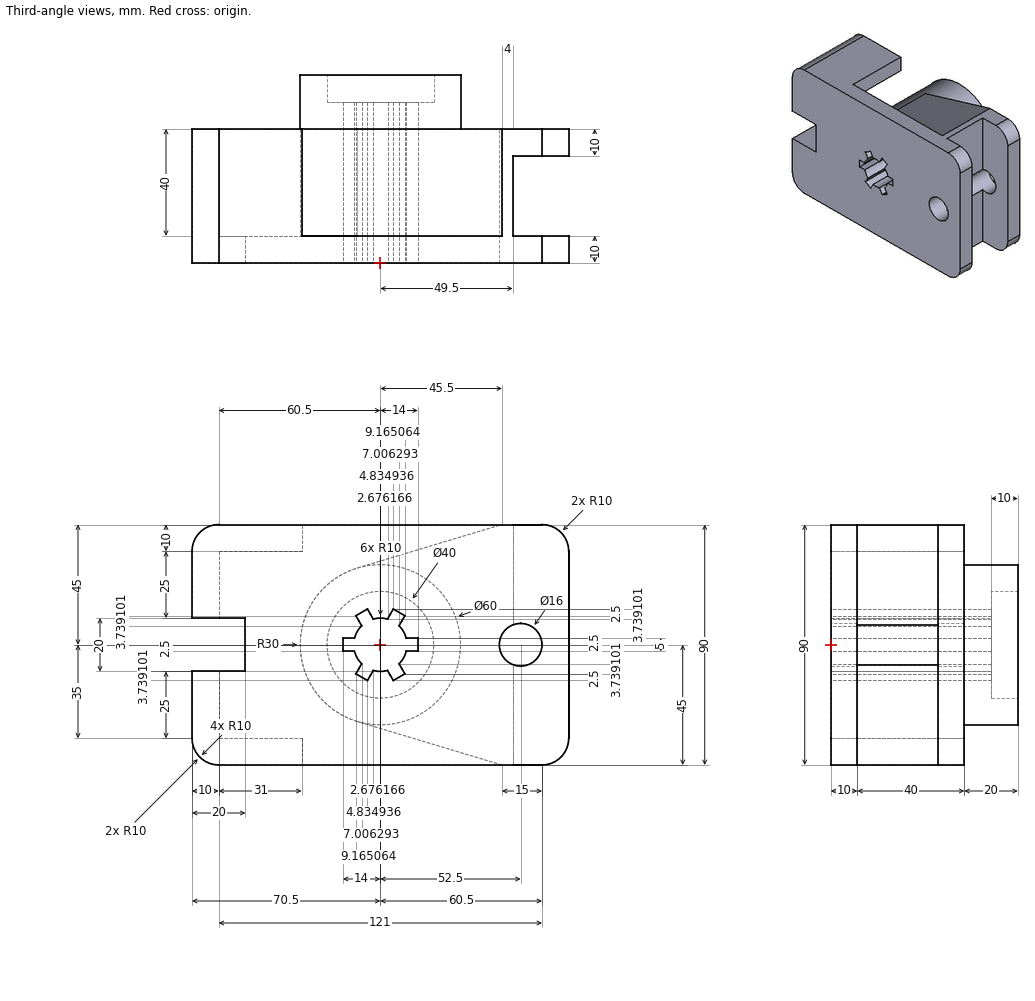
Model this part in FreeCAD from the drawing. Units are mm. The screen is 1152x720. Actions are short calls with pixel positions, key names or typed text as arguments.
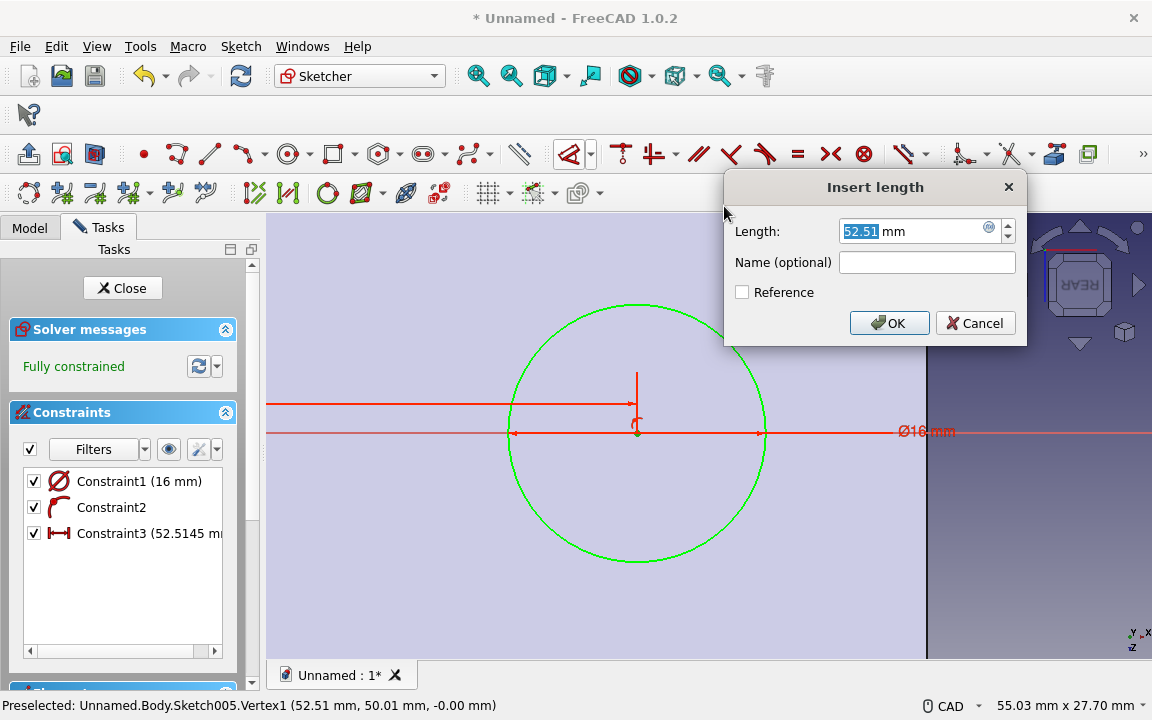
text(52.5)
key(Return)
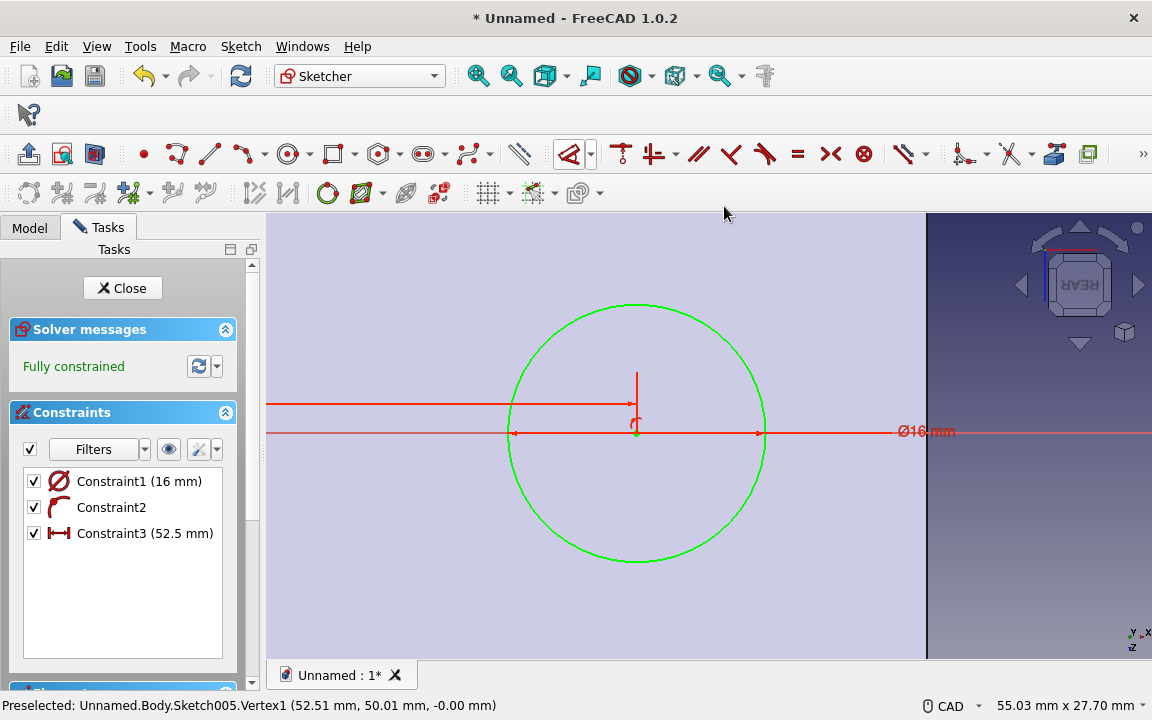
click(123, 288)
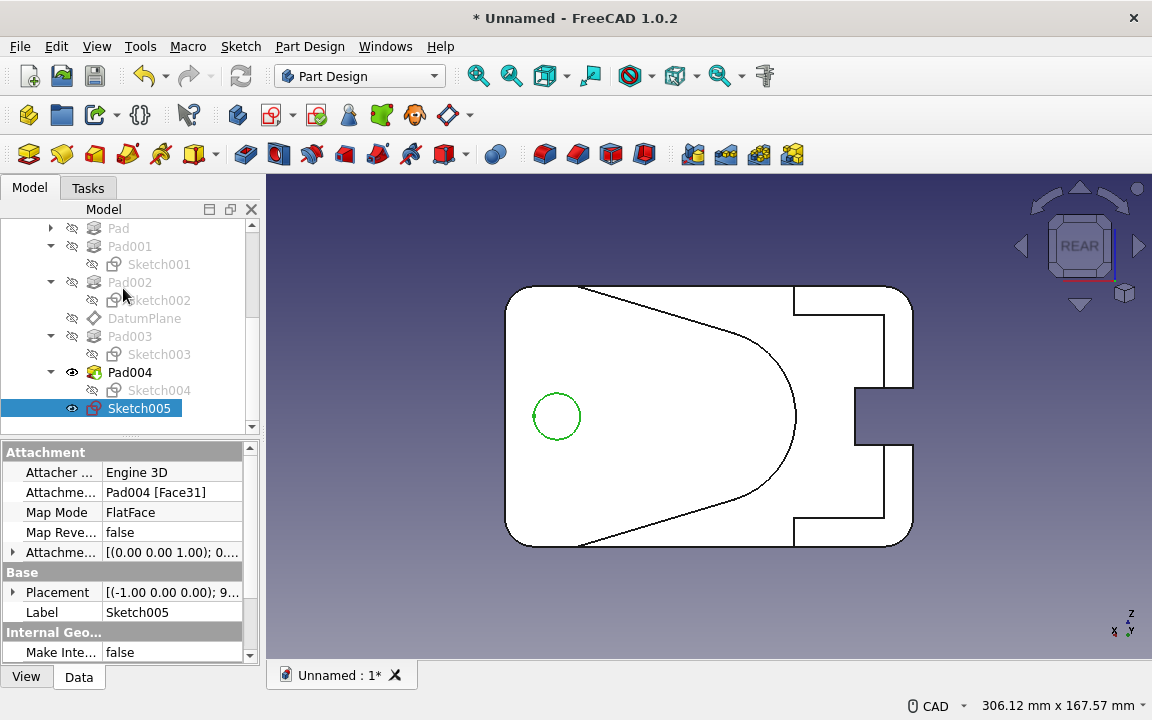
click(246, 154)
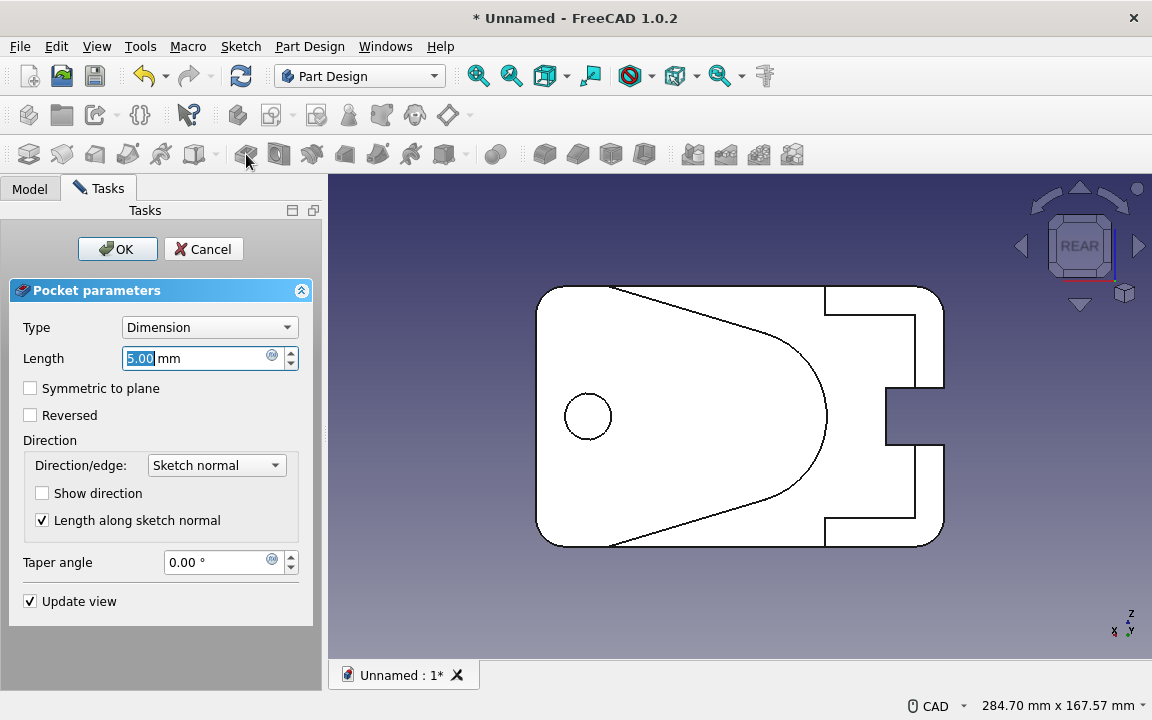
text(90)
key(Tab)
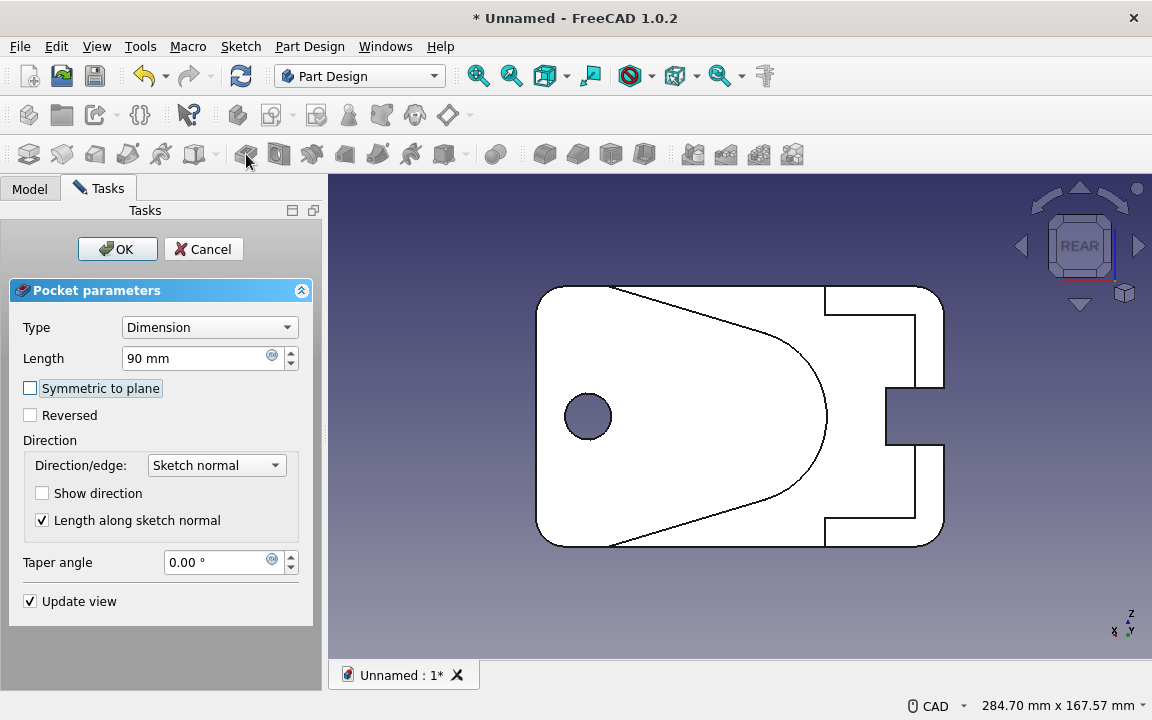
click(118, 249)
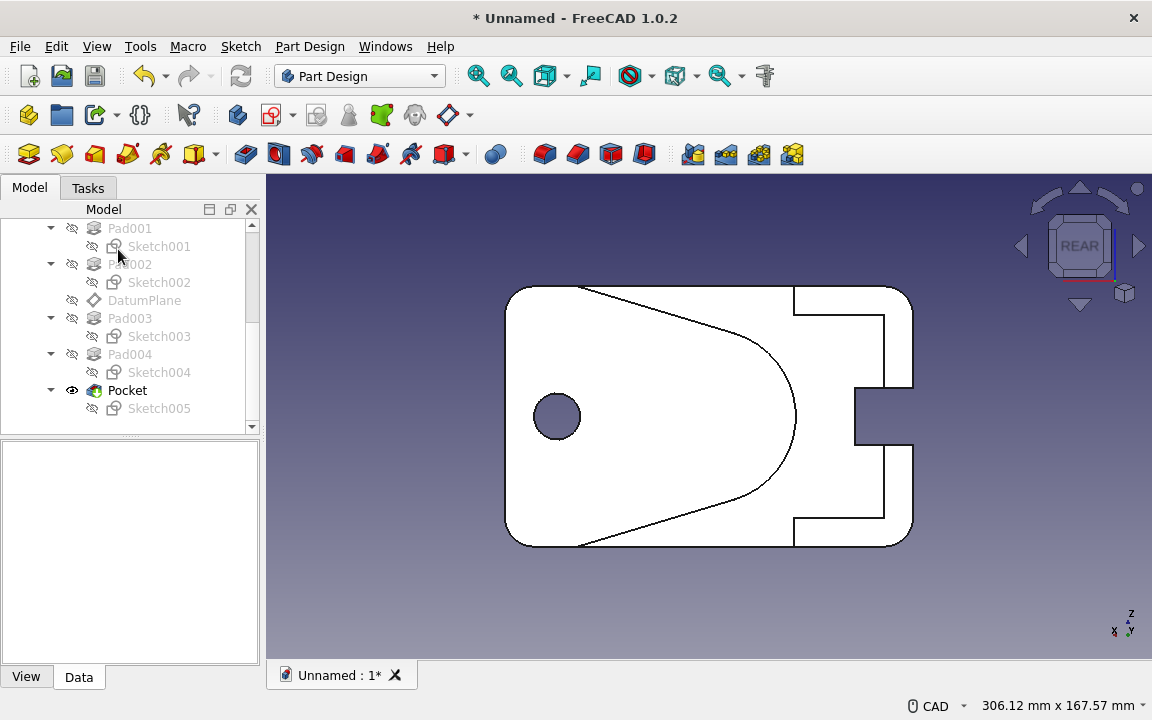
click(692, 416)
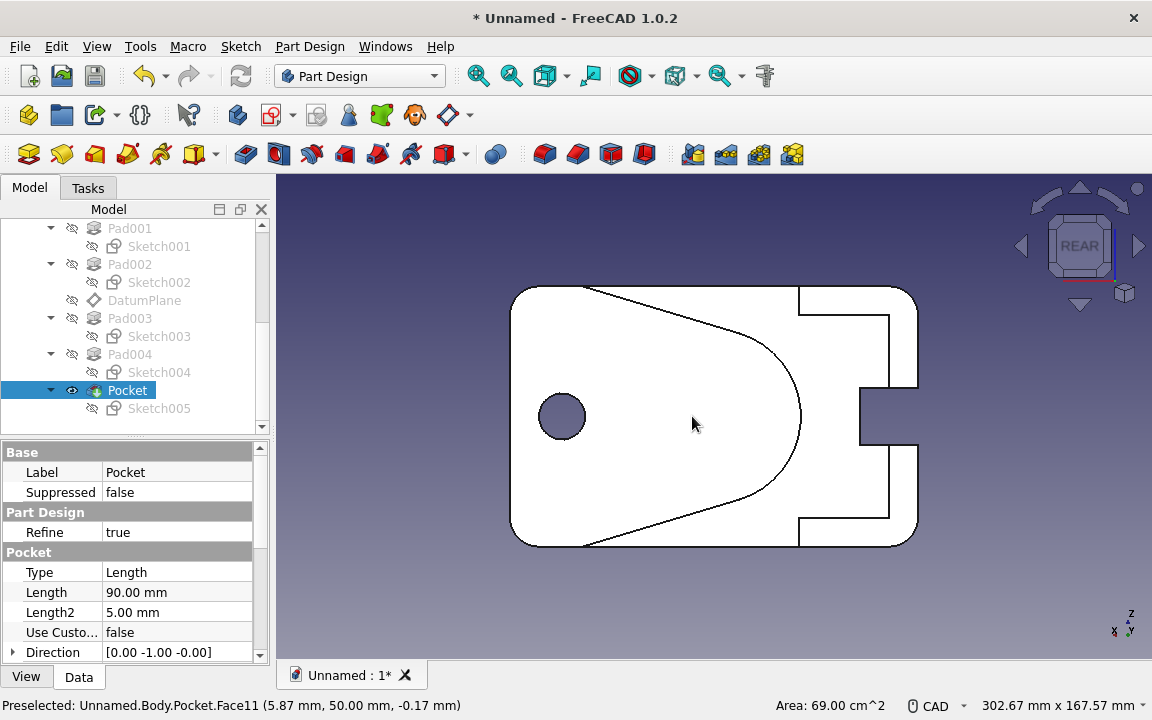
click(270, 116)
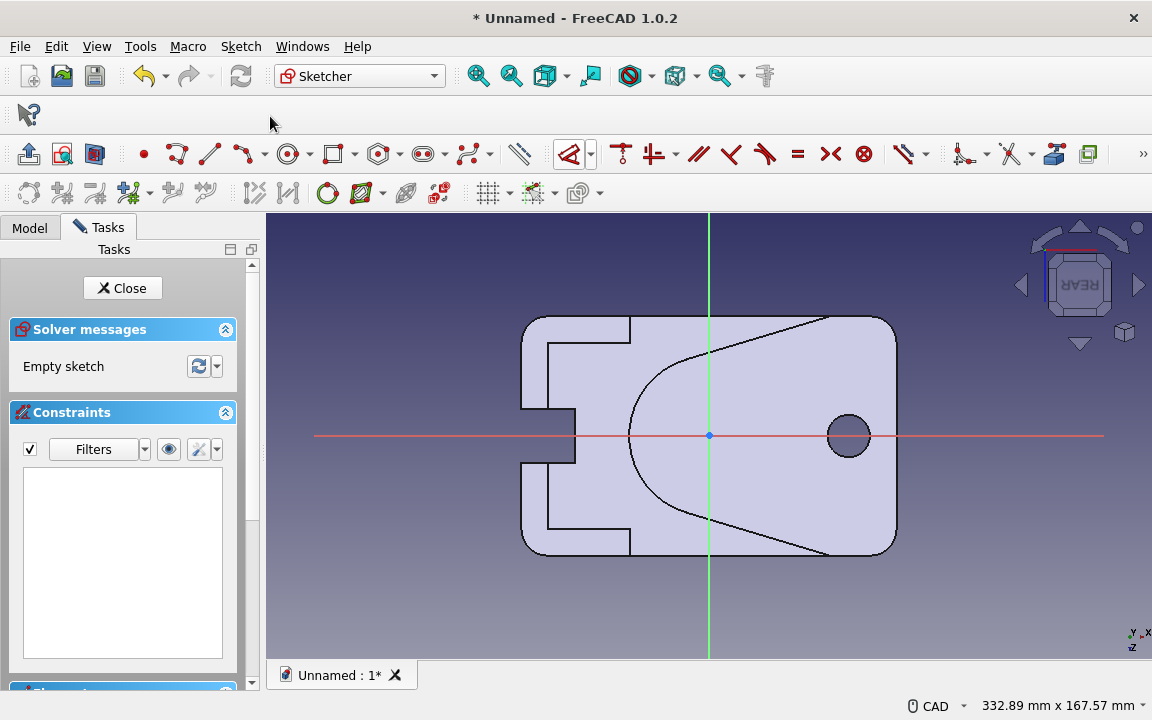
scroll(792, 436, up, 3)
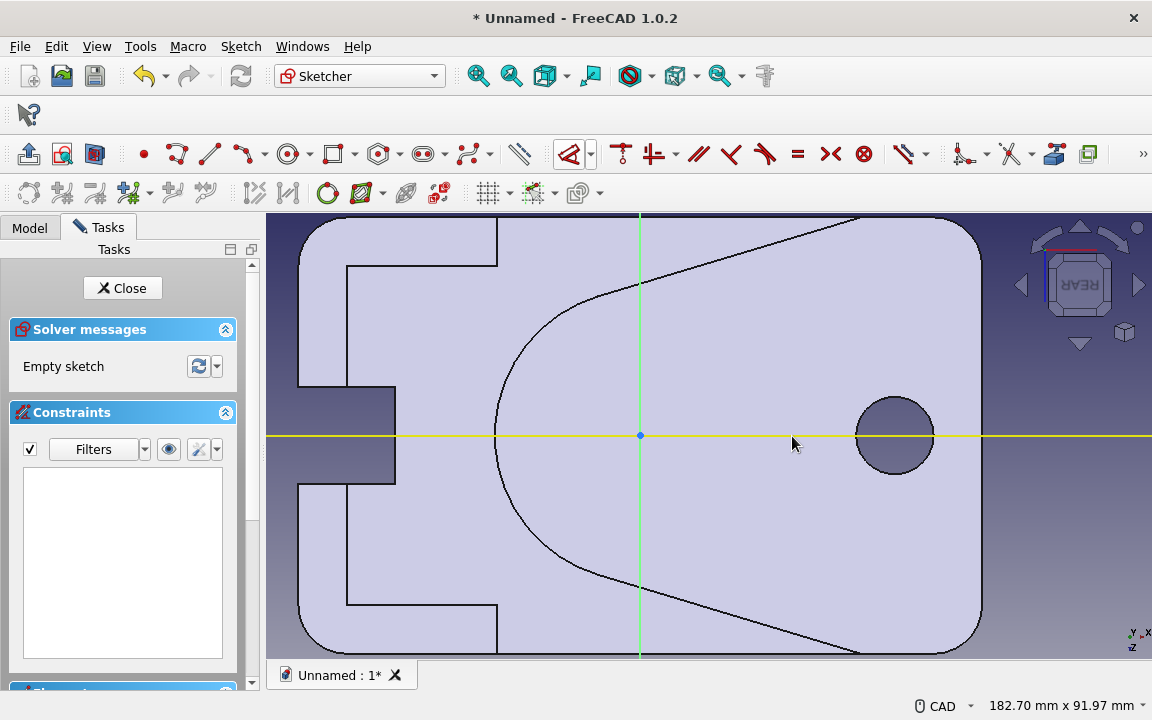
click(288, 154)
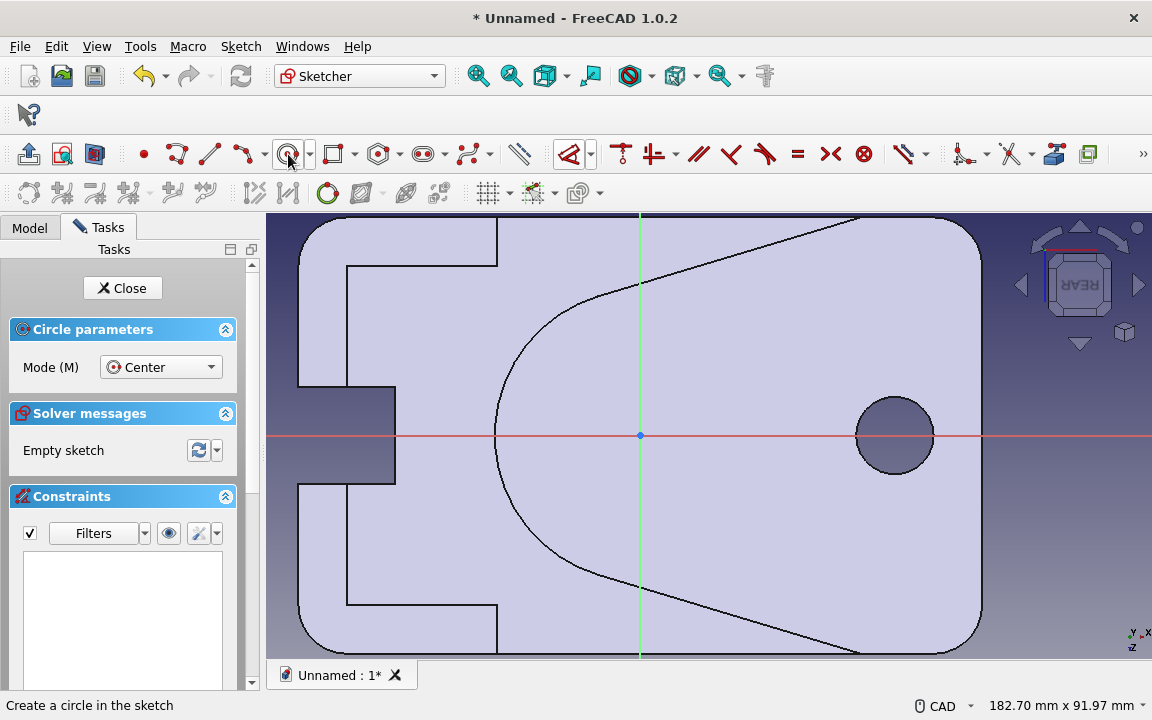
click(640, 436)
move(743, 333)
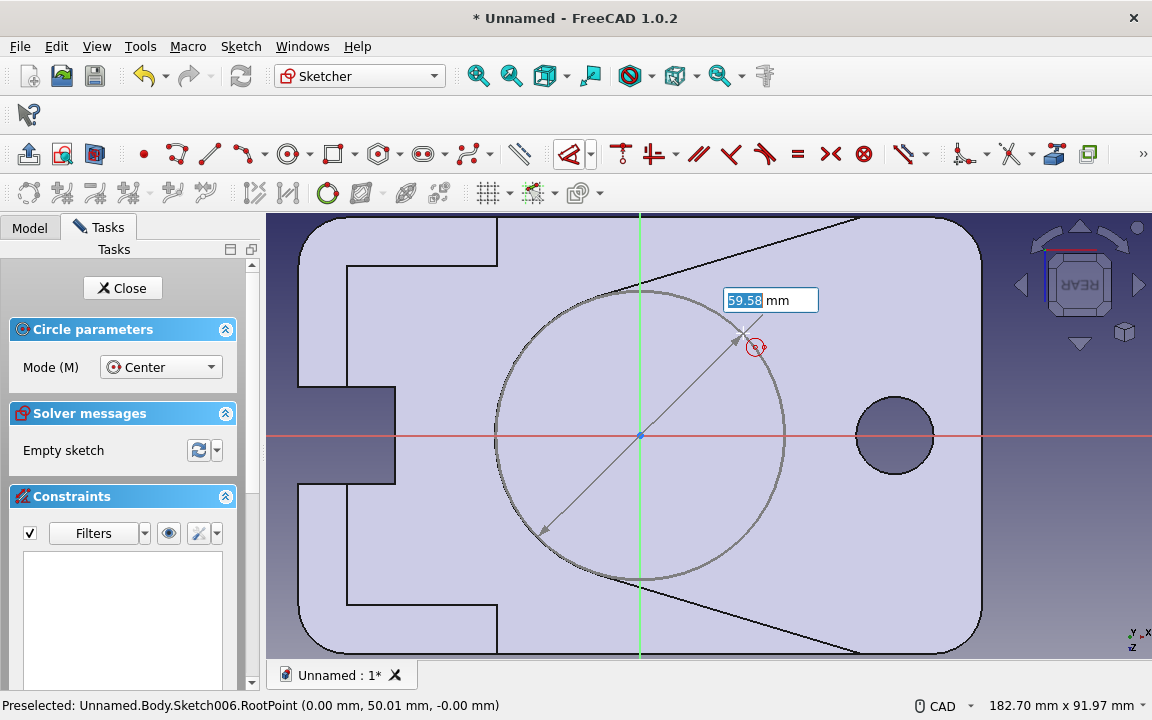
text(60)
key(Return)
key(Escape)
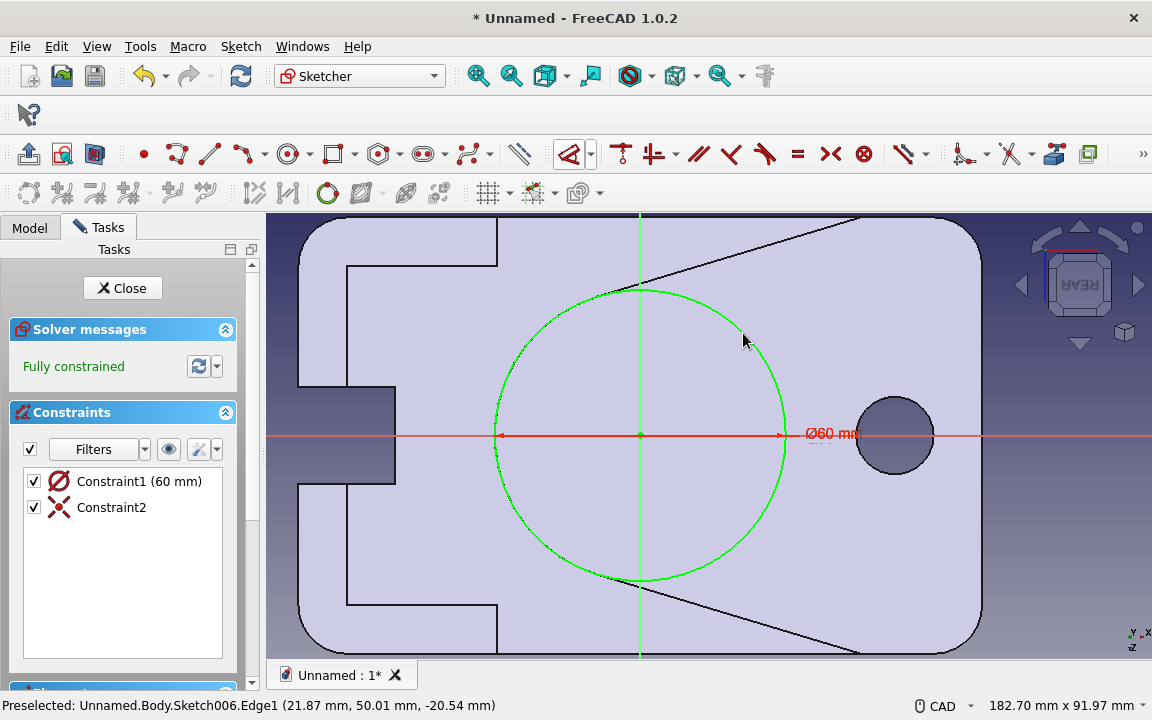
click(123, 288)